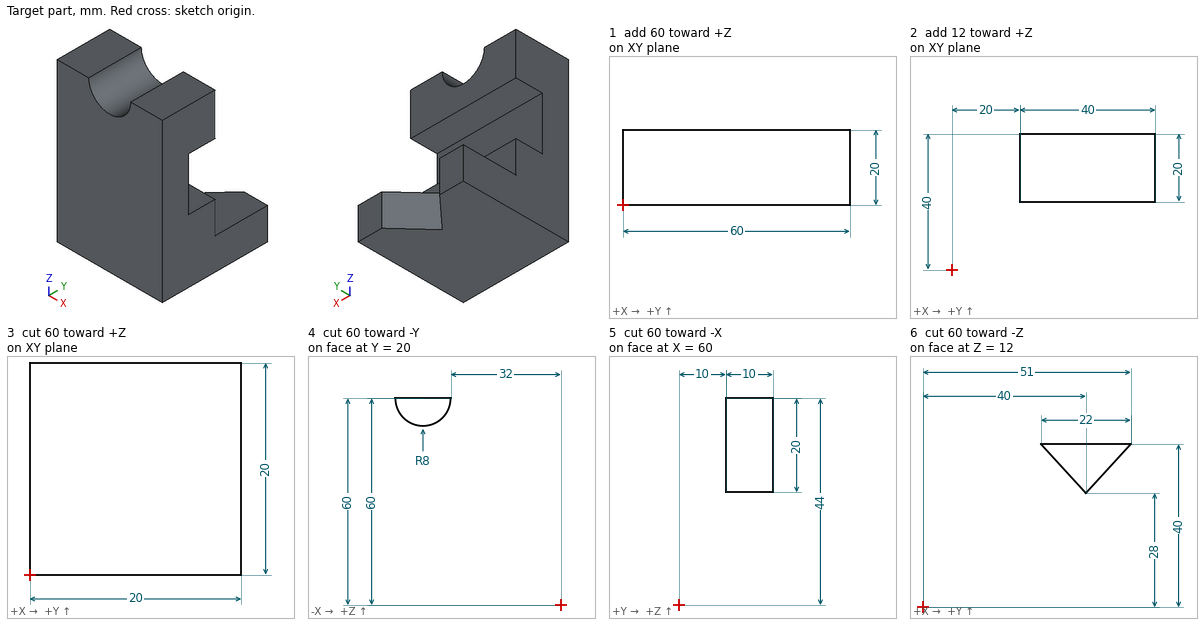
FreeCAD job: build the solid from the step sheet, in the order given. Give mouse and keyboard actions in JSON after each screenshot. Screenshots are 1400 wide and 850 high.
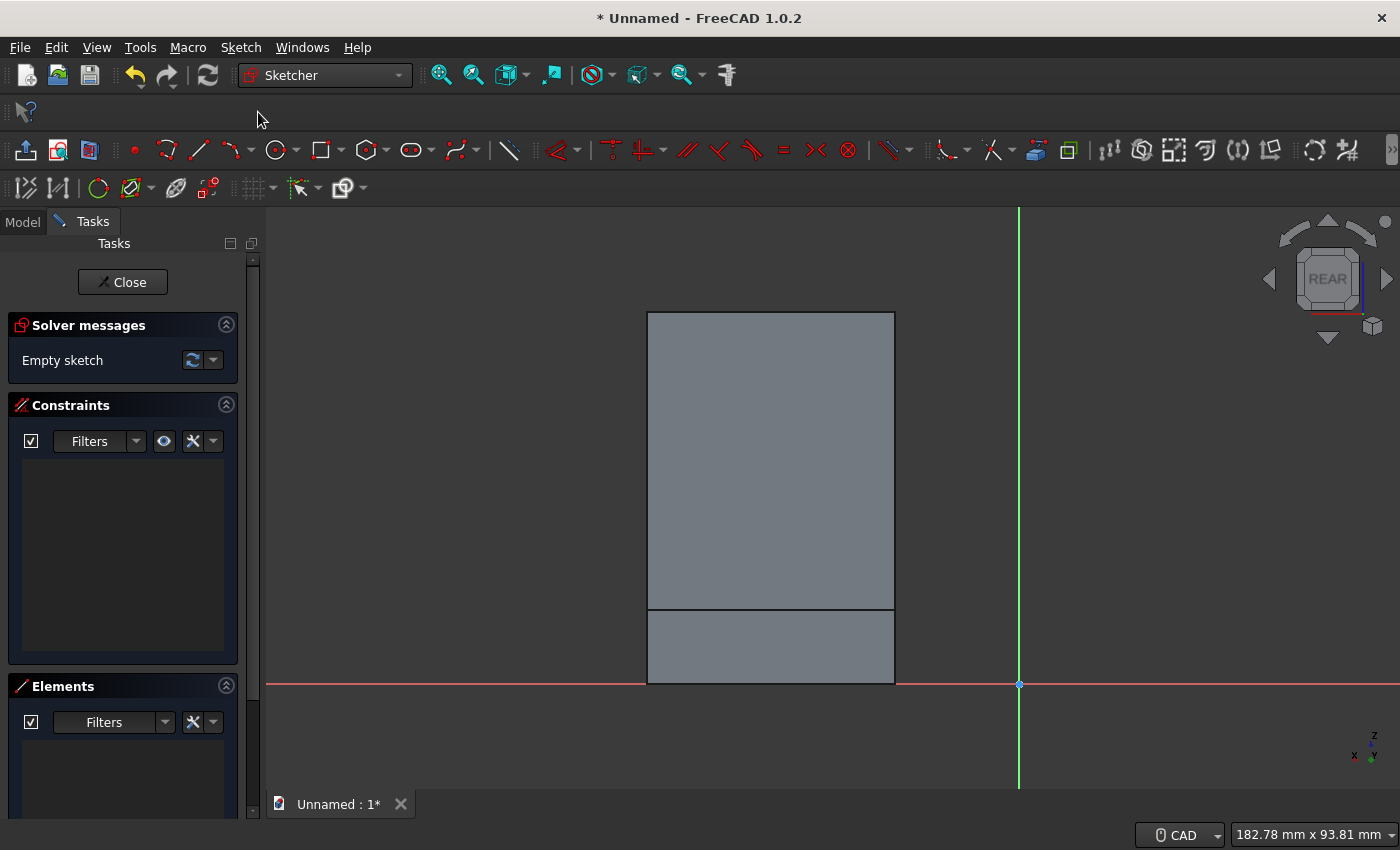
{"action": "scroll", "coordinate": [772, 311], "scroll_direction": "up", "scroll_amount": 10}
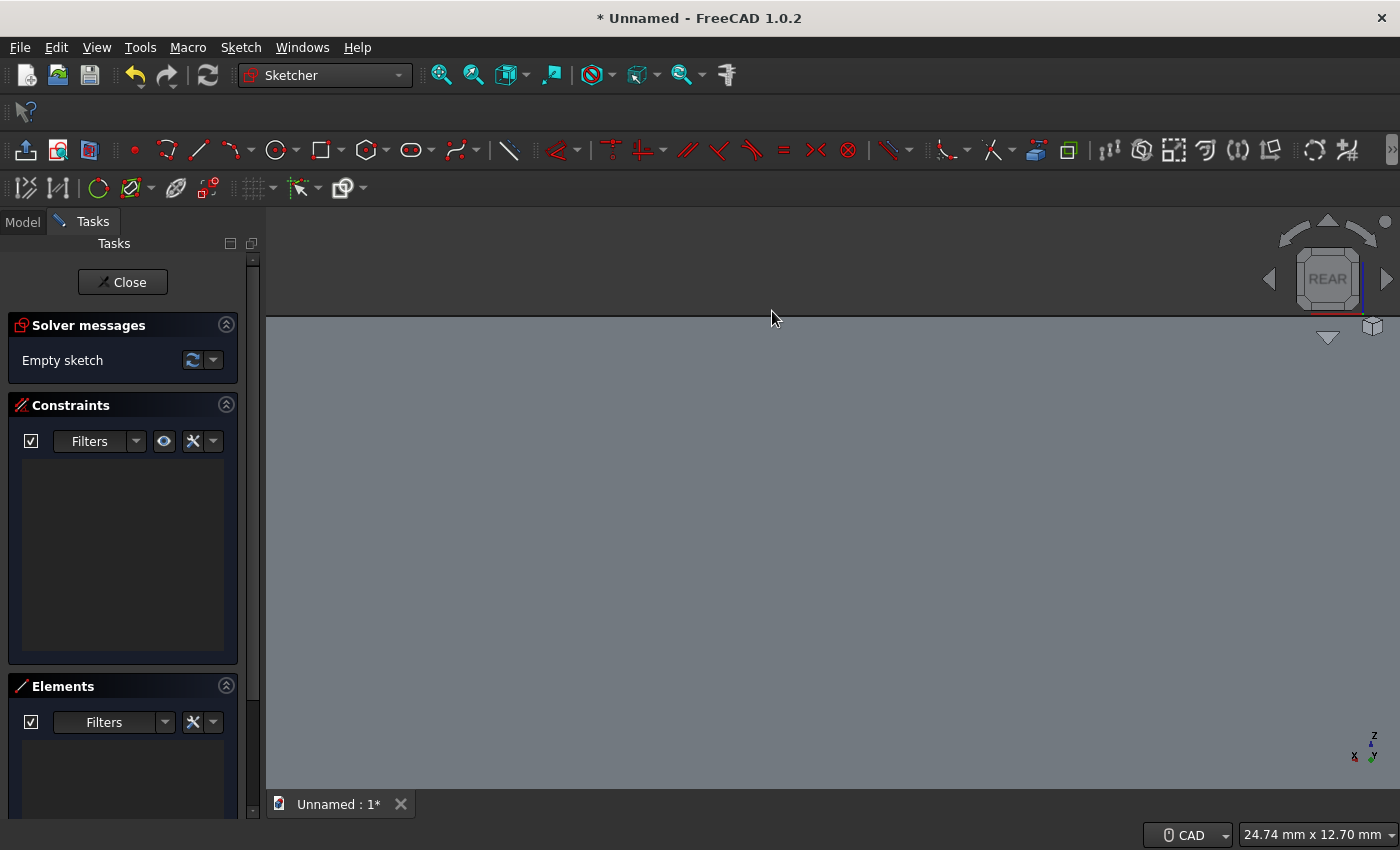
{"action": "left_click", "coordinate": [200, 150]}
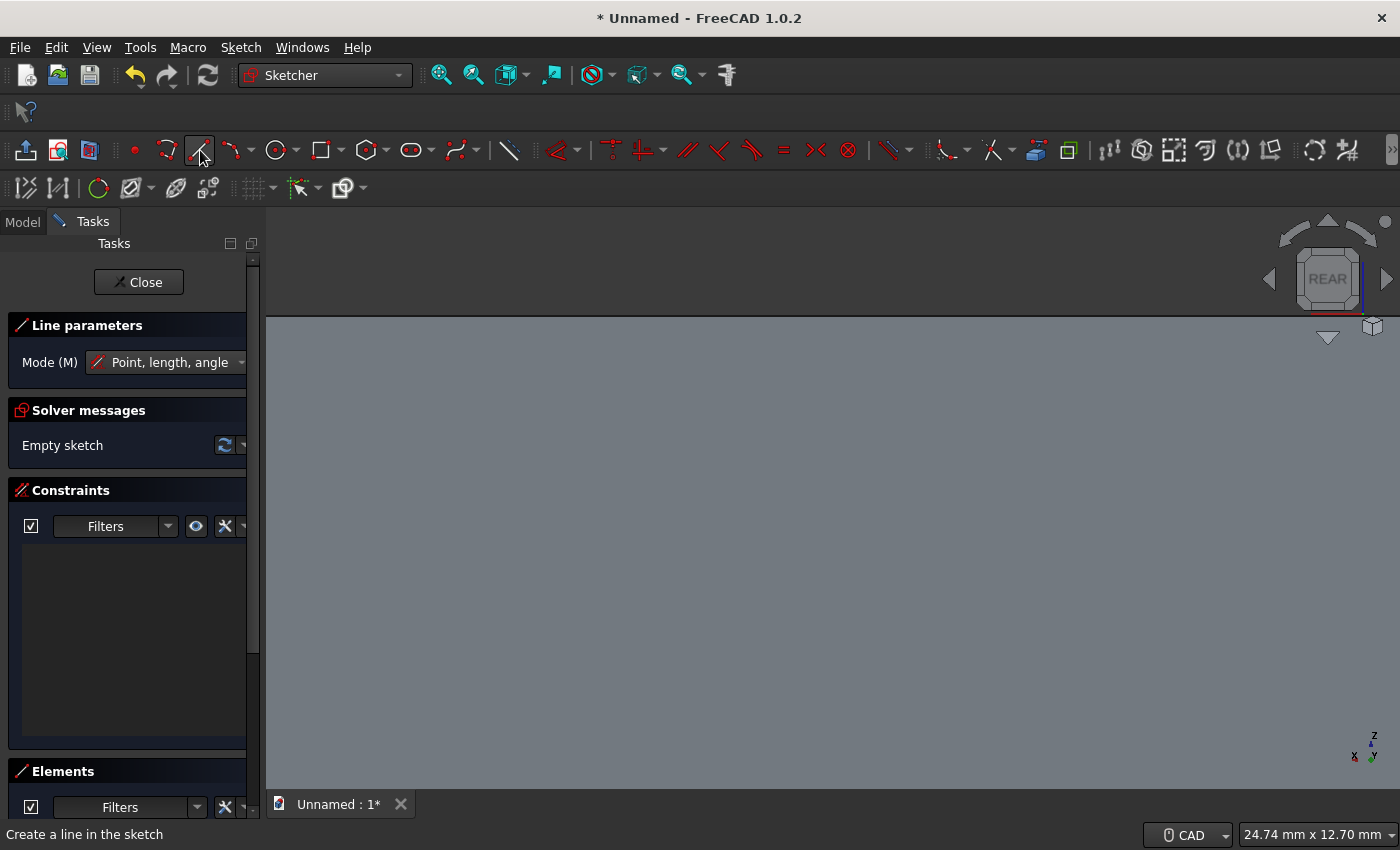
{"action": "left_click", "coordinate": [1128, 316]}
{"action": "left_click", "coordinate": [395, 316]}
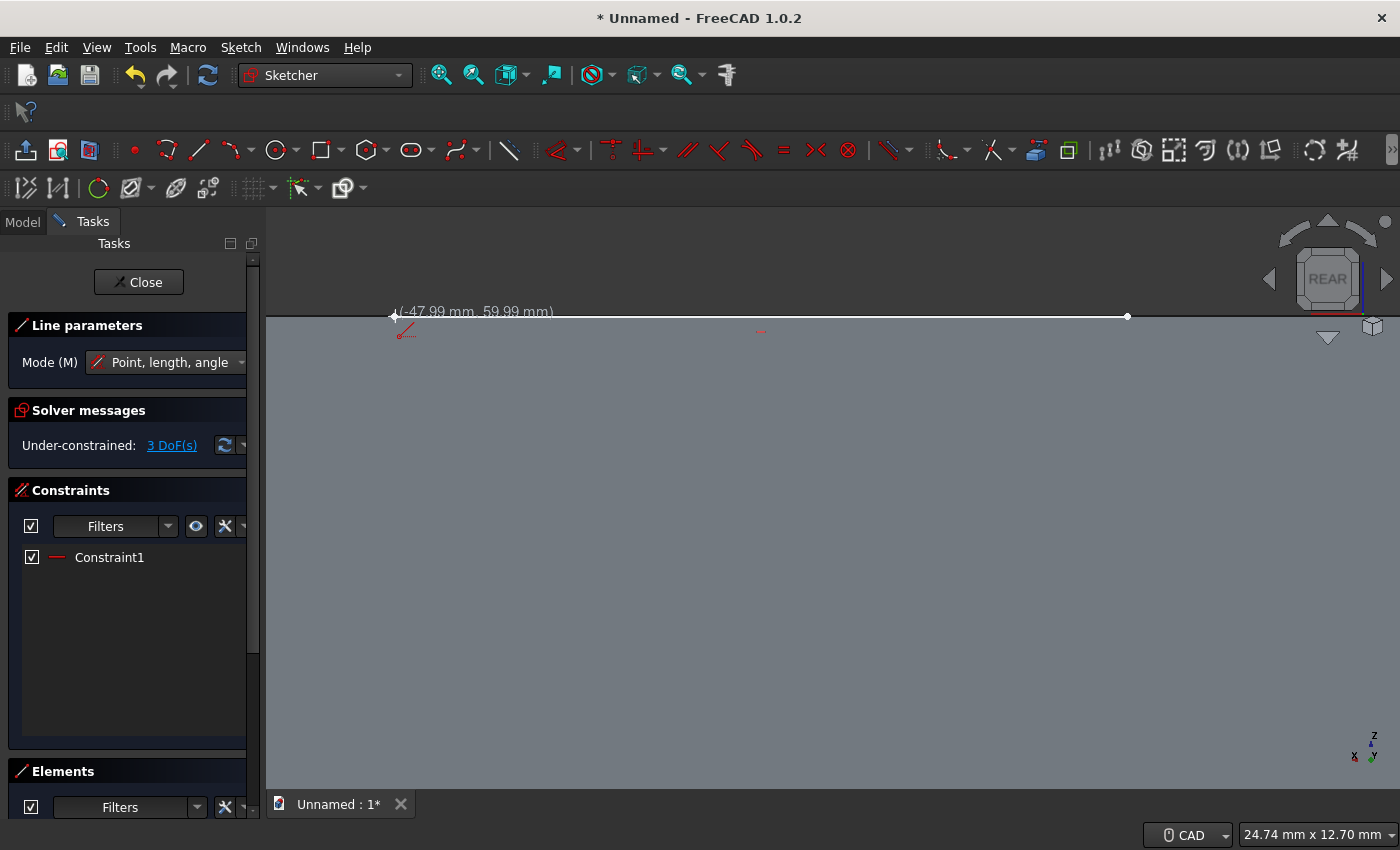
{"action": "left_click", "coordinate": [232, 150]}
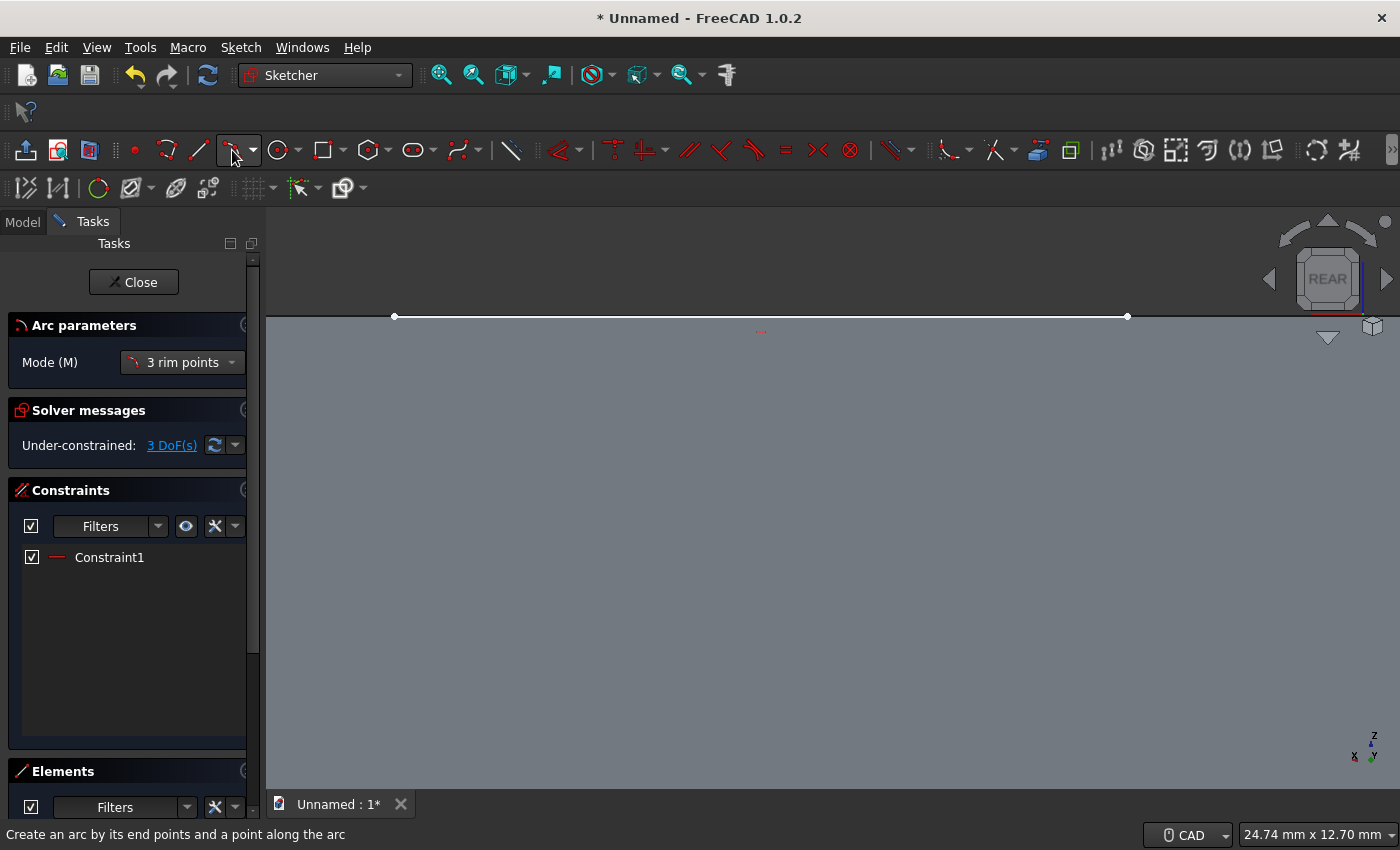
{"action": "left_click", "coordinate": [395, 317]}
{"action": "left_click", "coordinate": [1128, 317]}
{"action": "left_click", "coordinate": [761, 683]}
{"action": "key", "text": "Escape"}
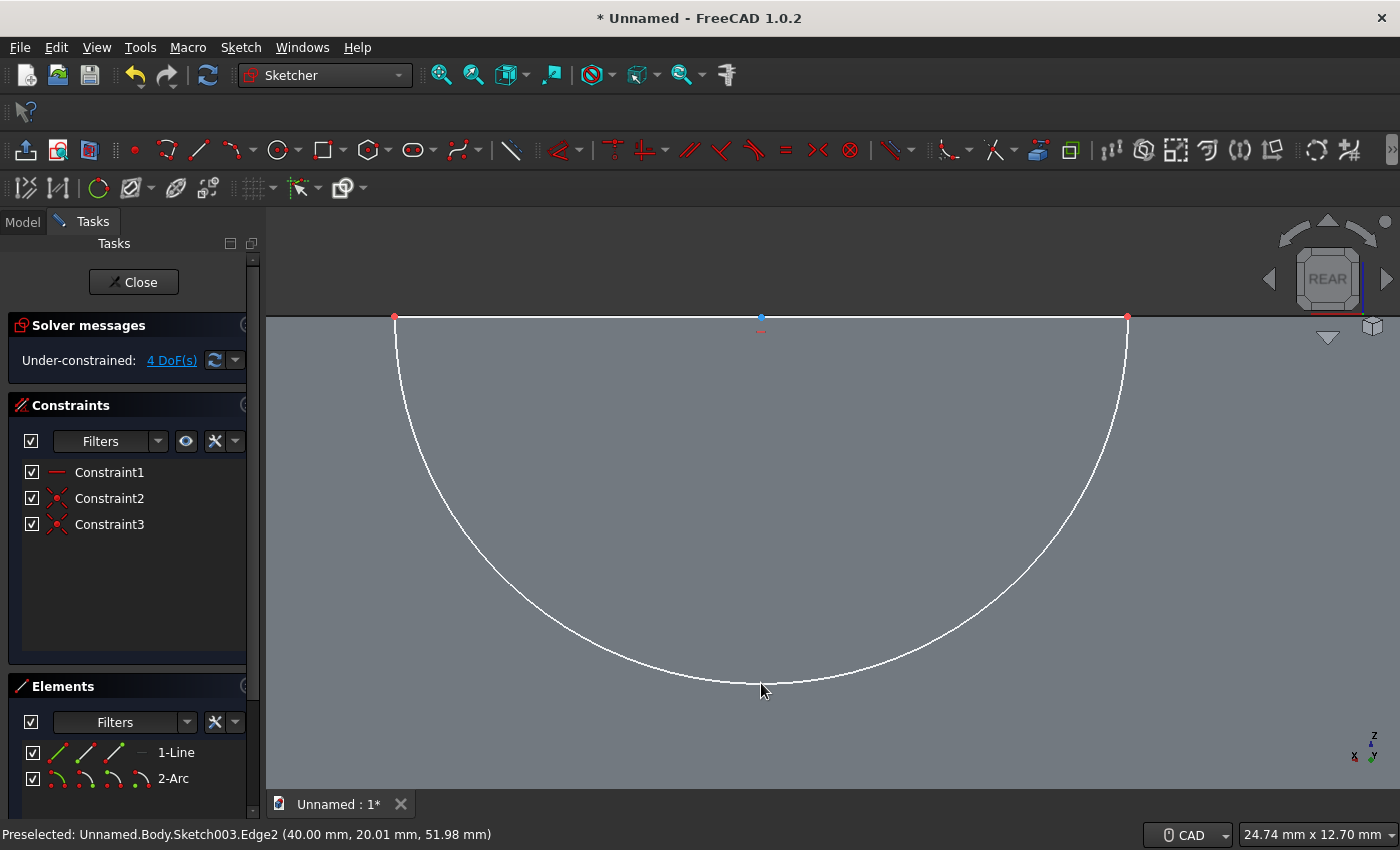
{"action": "key", "text": "d"}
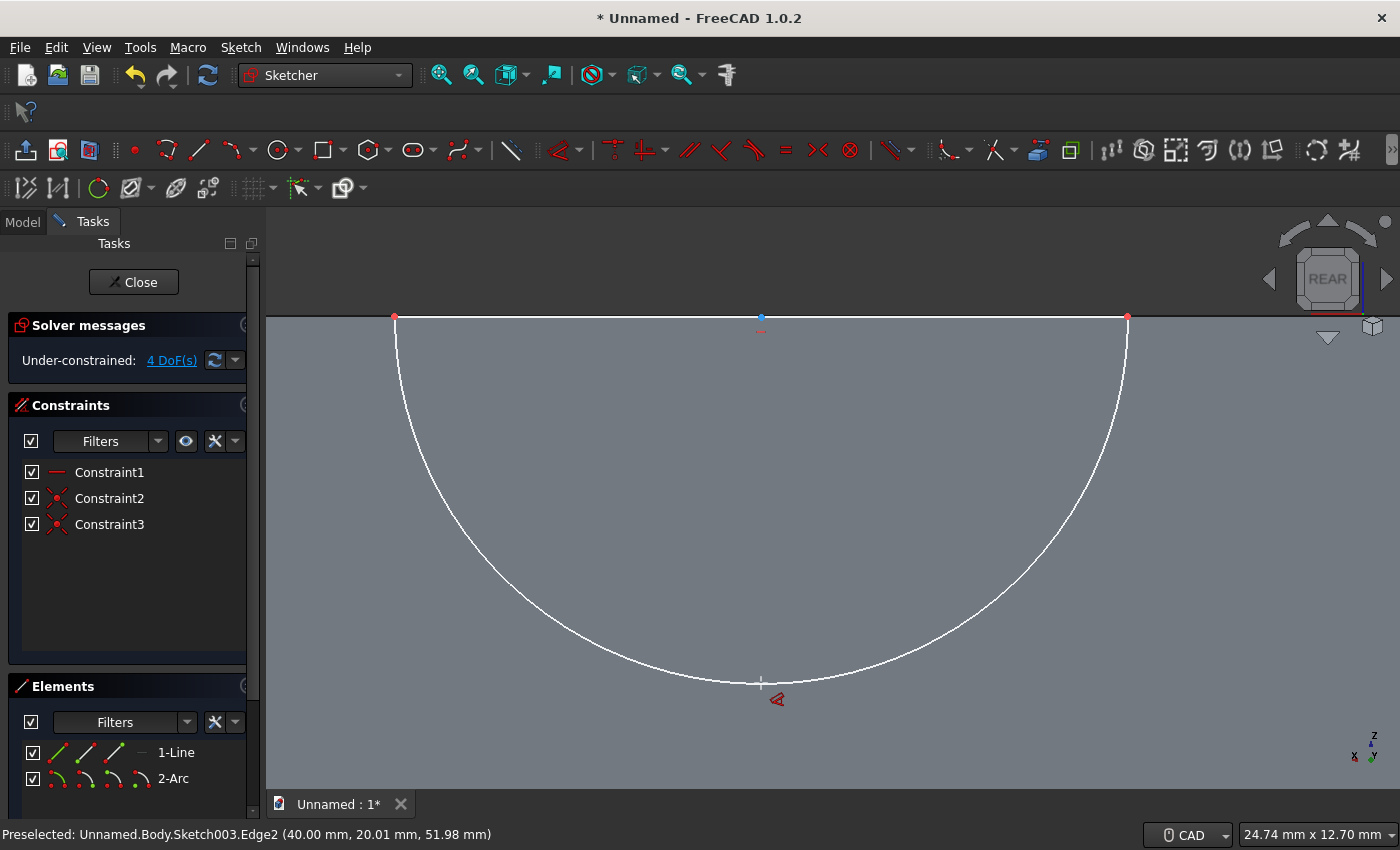
{"action": "left_click", "coordinate": [546, 614]}
{"action": "left_click", "coordinate": [527, 640]}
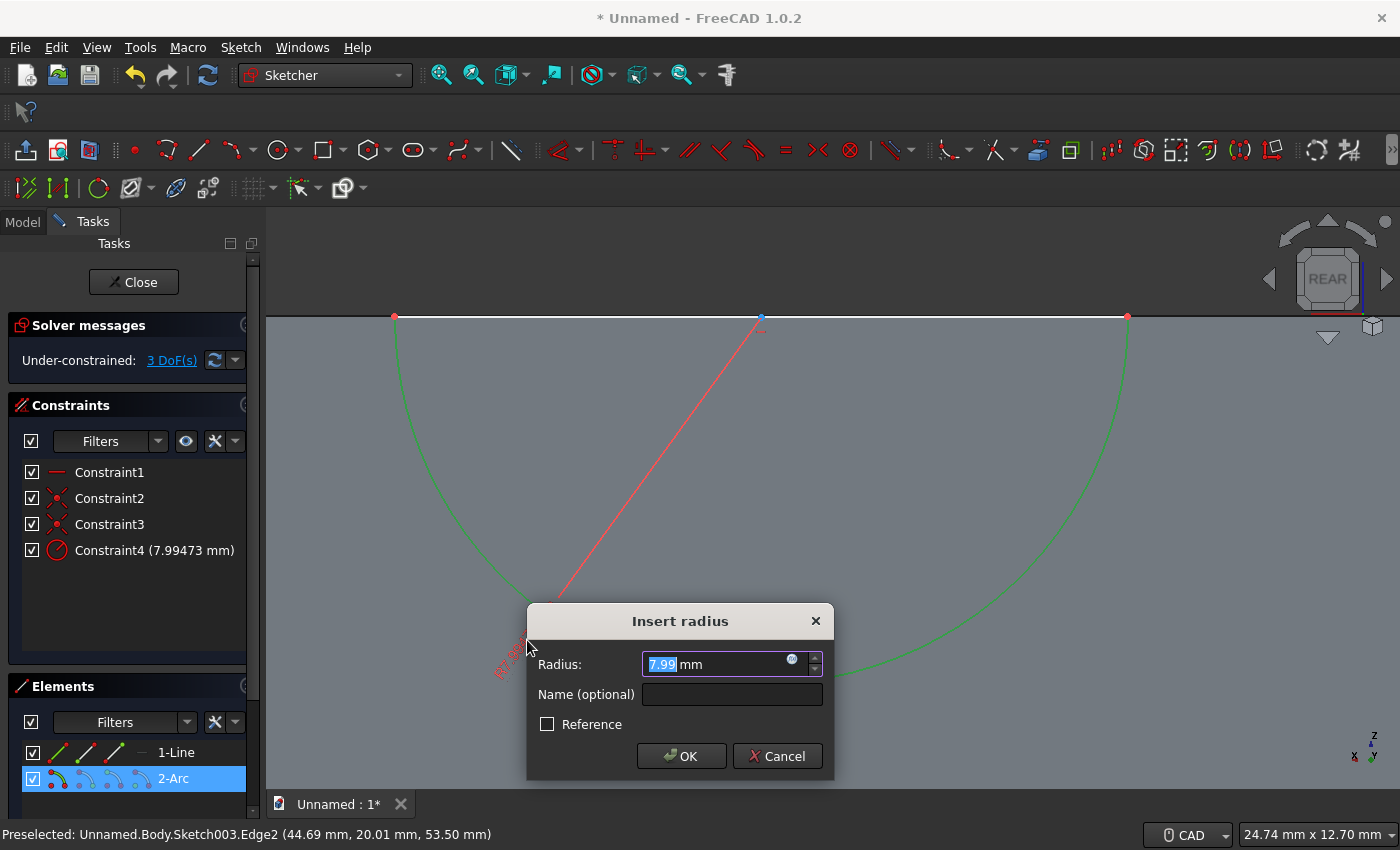
{"action": "type", "text": "8"}
{"action": "key", "text": "Return"}